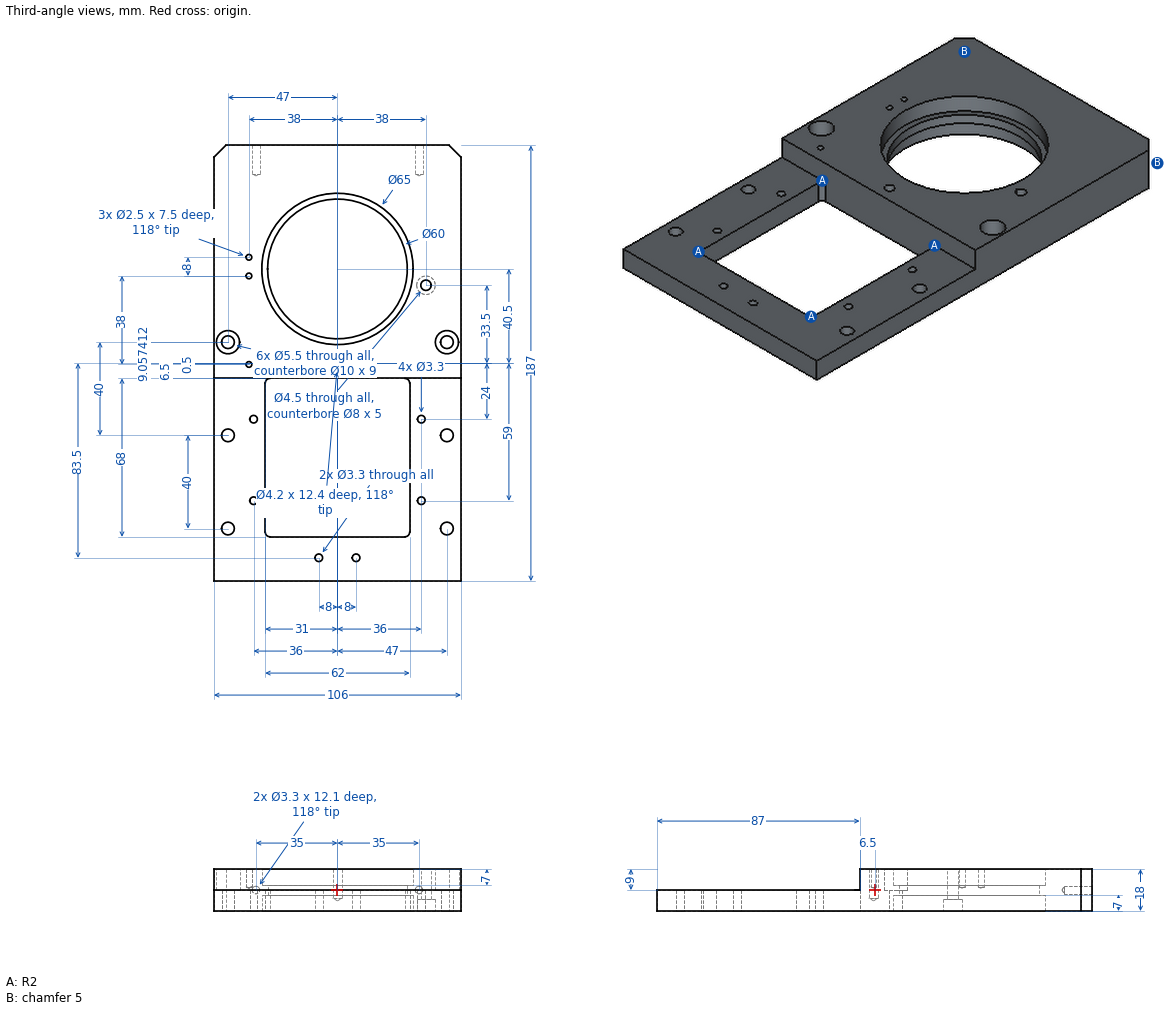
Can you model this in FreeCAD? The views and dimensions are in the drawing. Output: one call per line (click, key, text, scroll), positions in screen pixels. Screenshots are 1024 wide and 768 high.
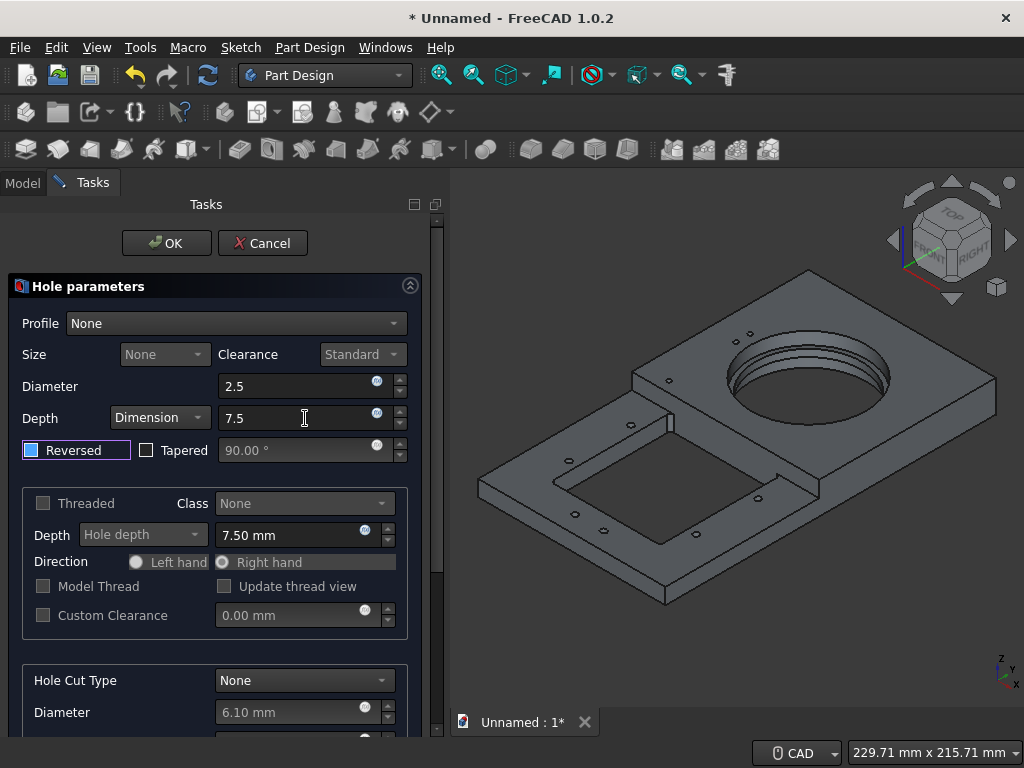
click(167, 243)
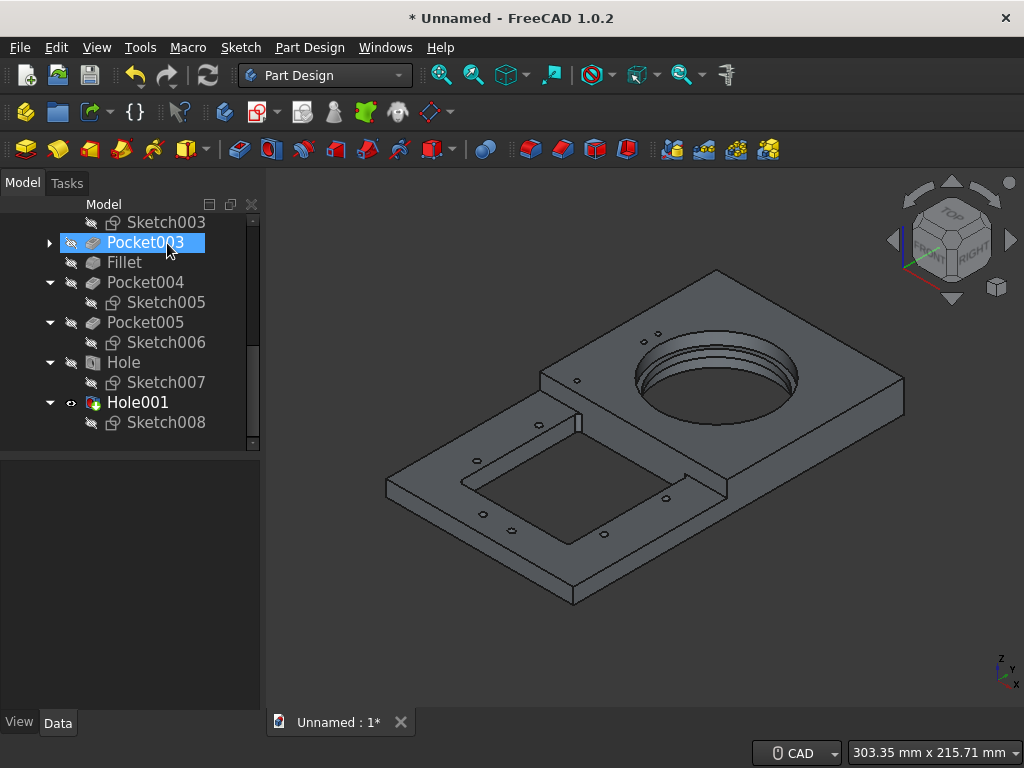
key(2)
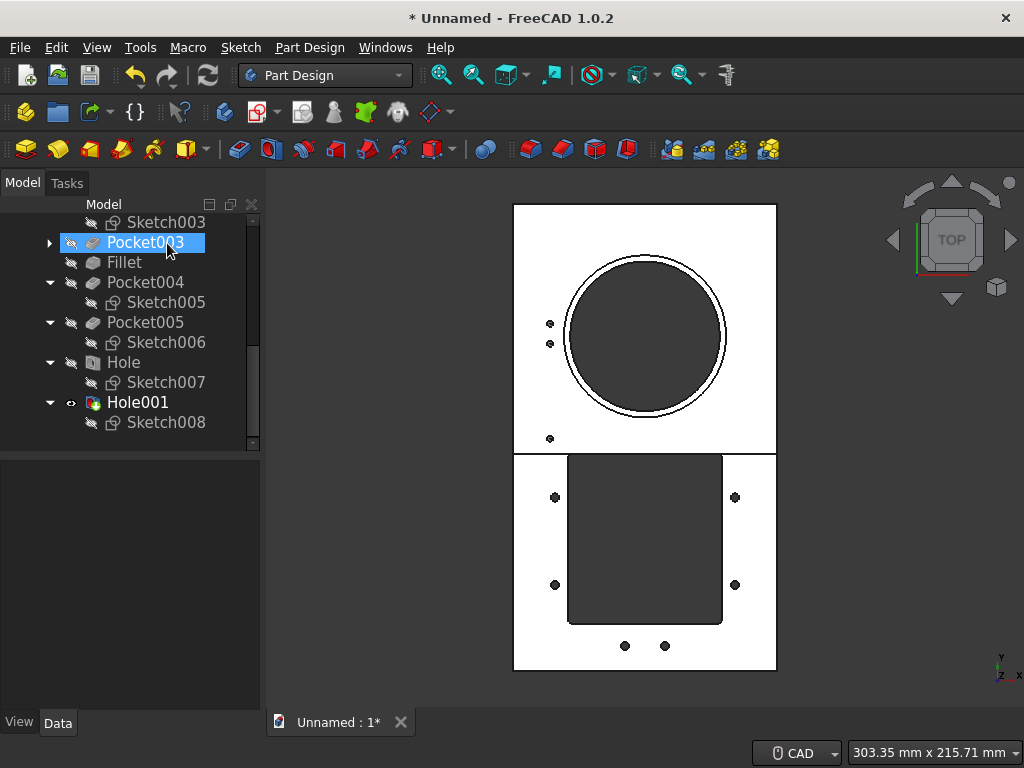
key(0)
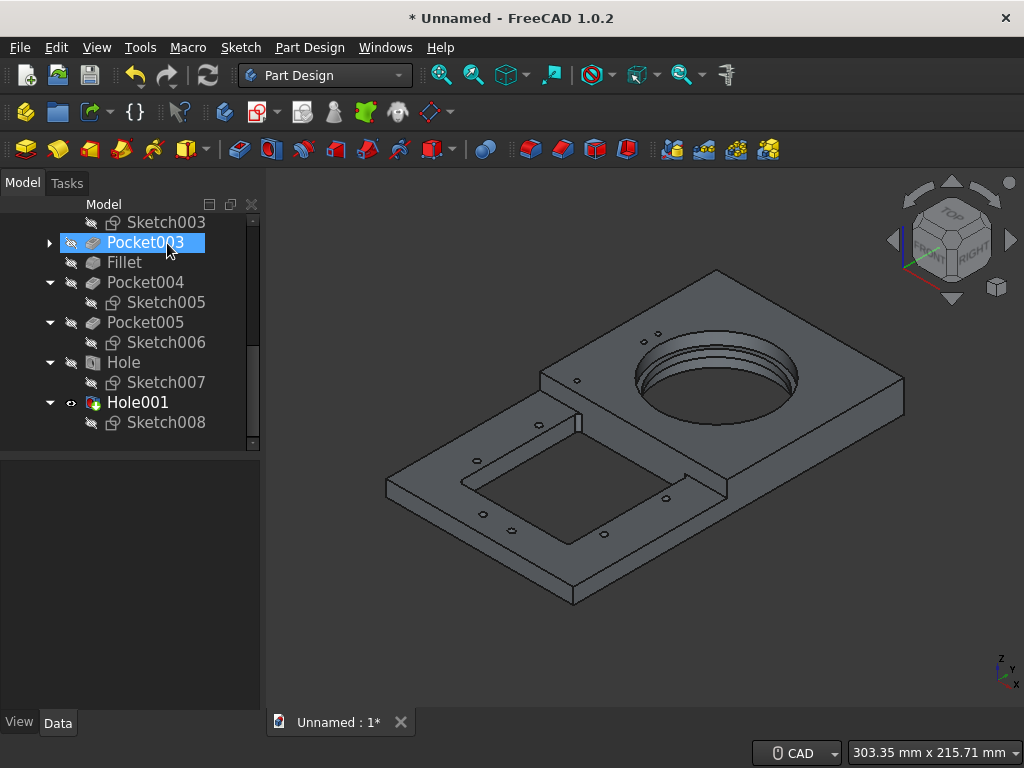
key(1)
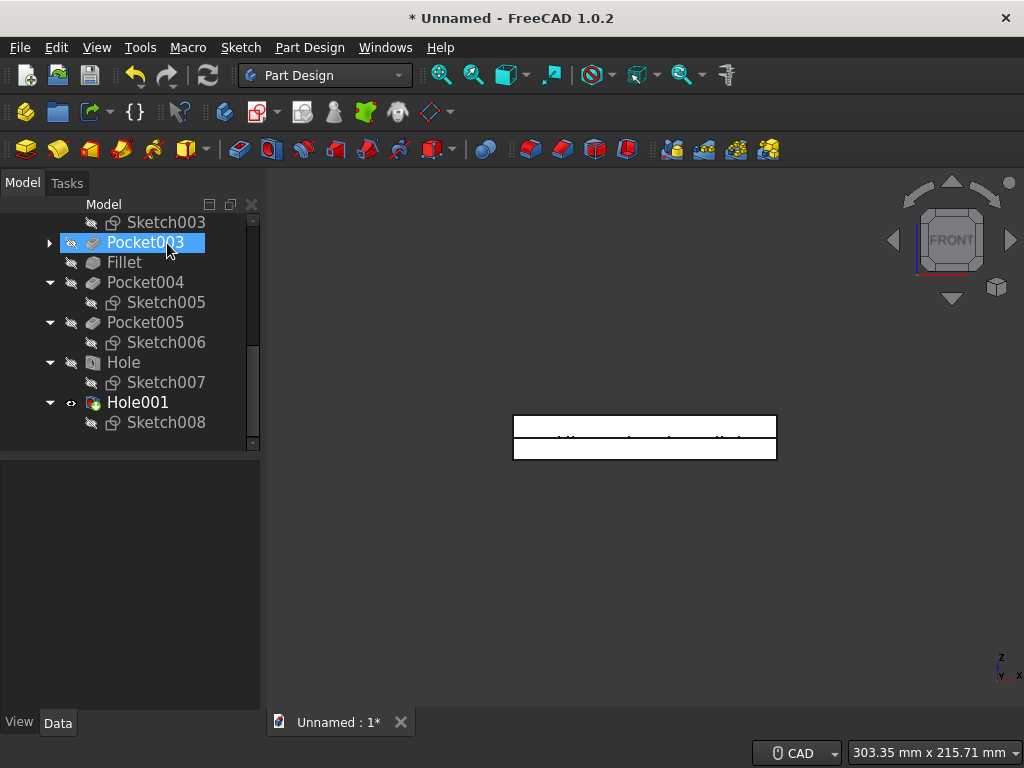
click(442, 76)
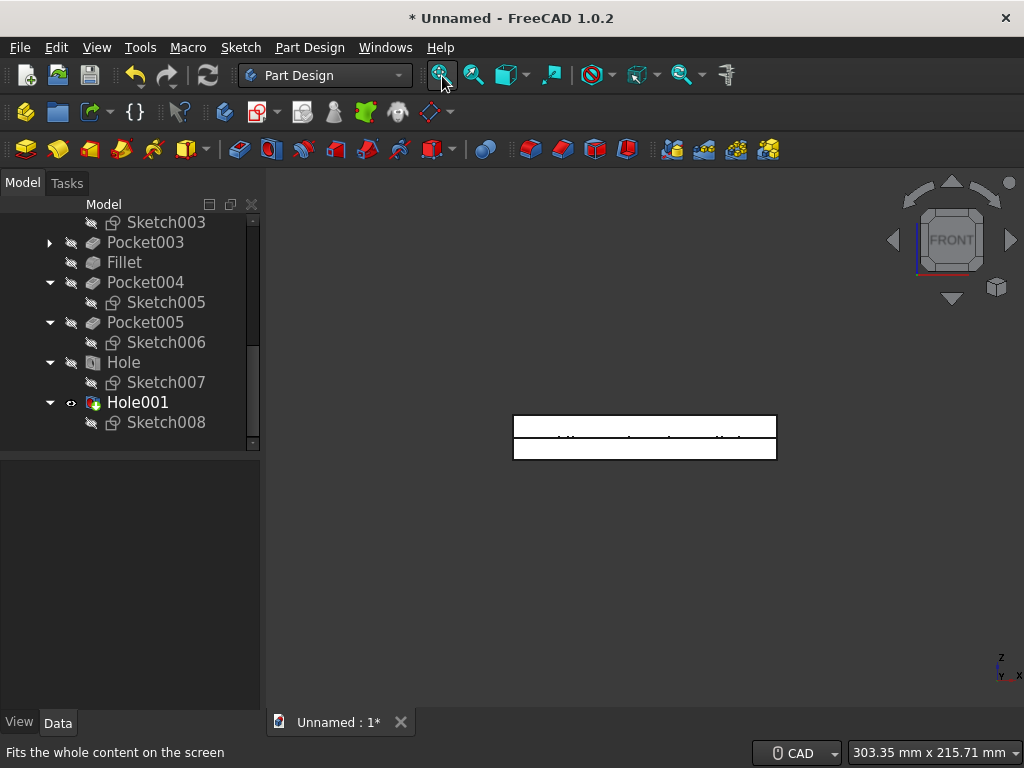
key(3)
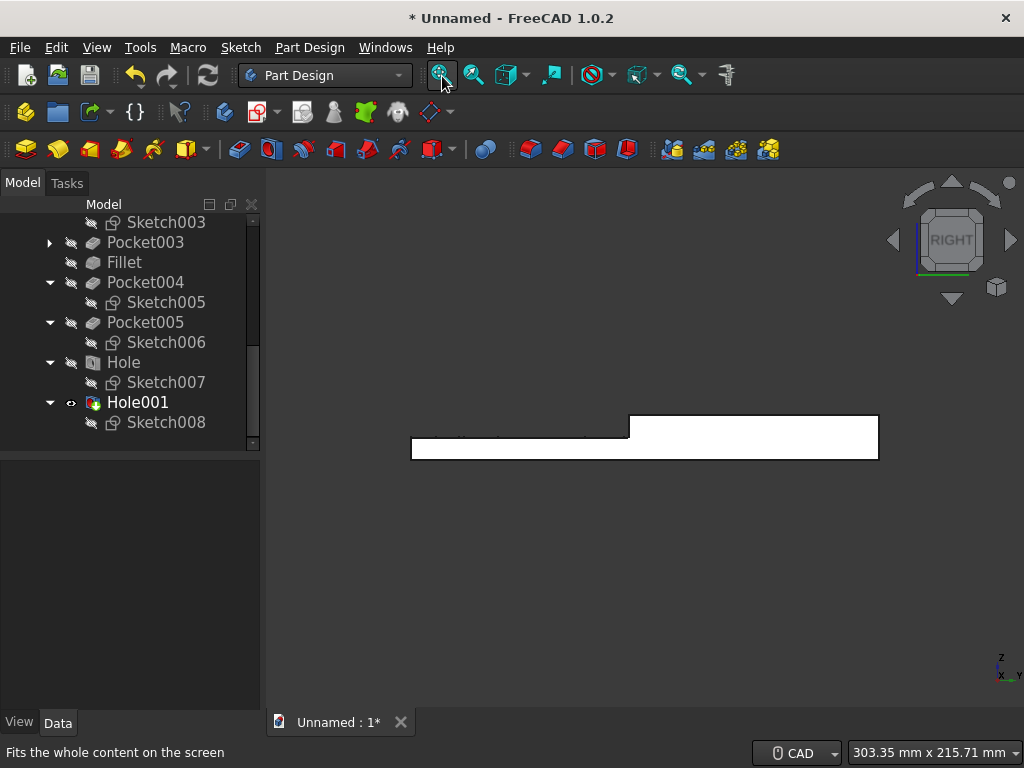
click(879, 436)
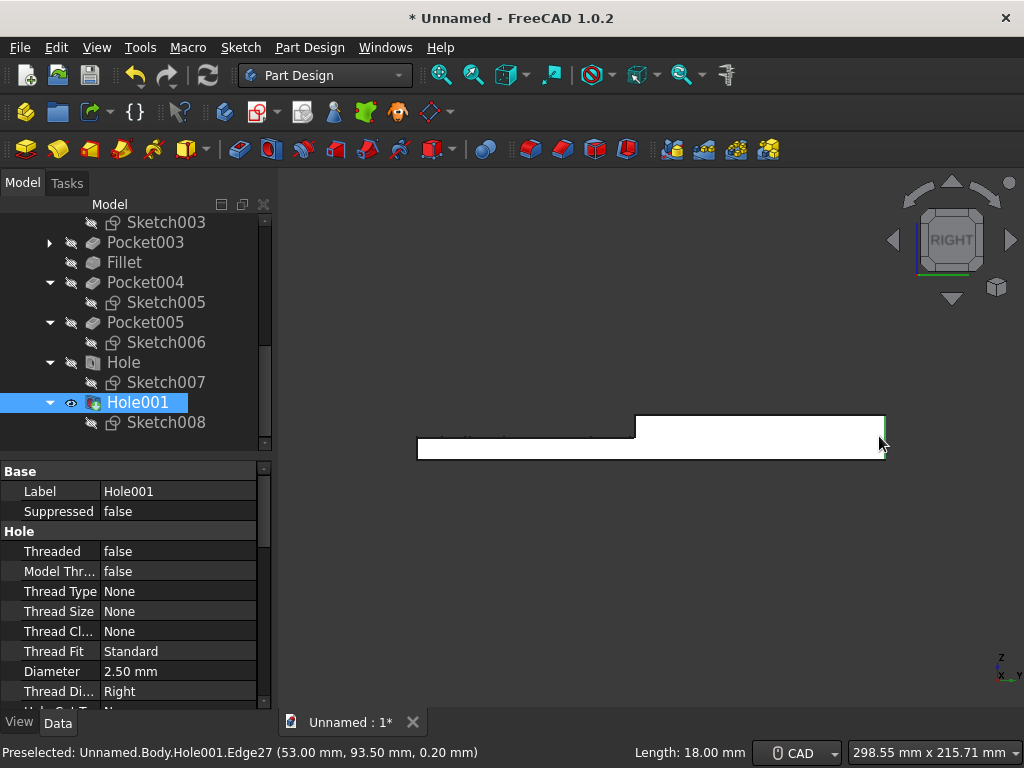
key(5)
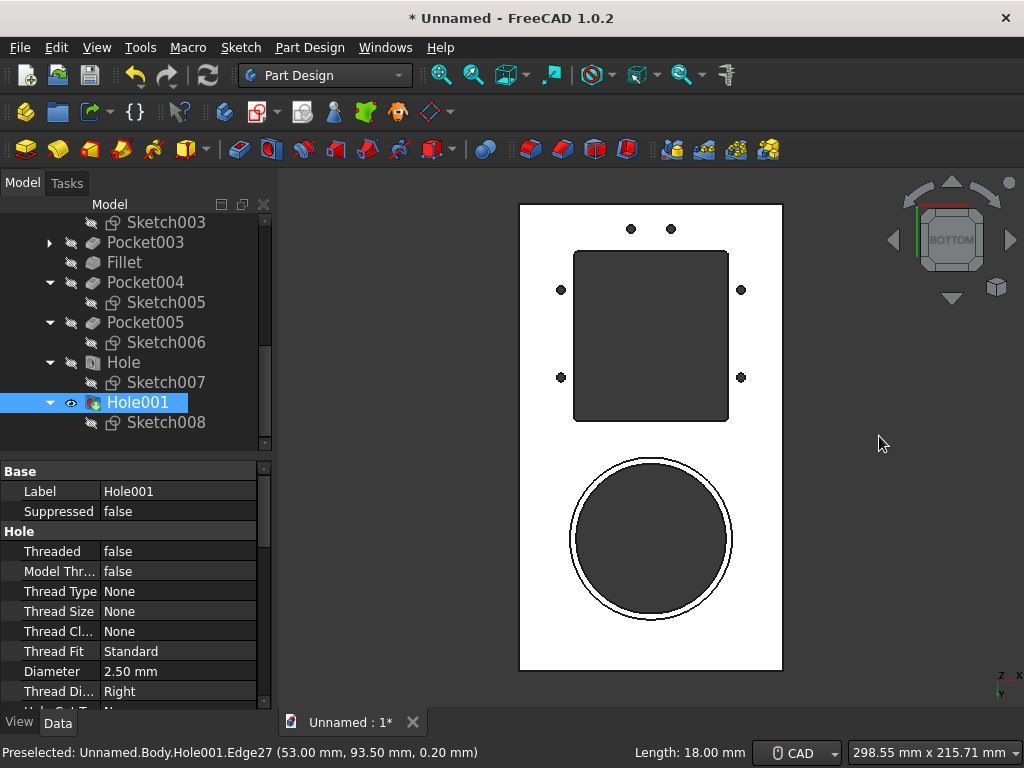
key(4)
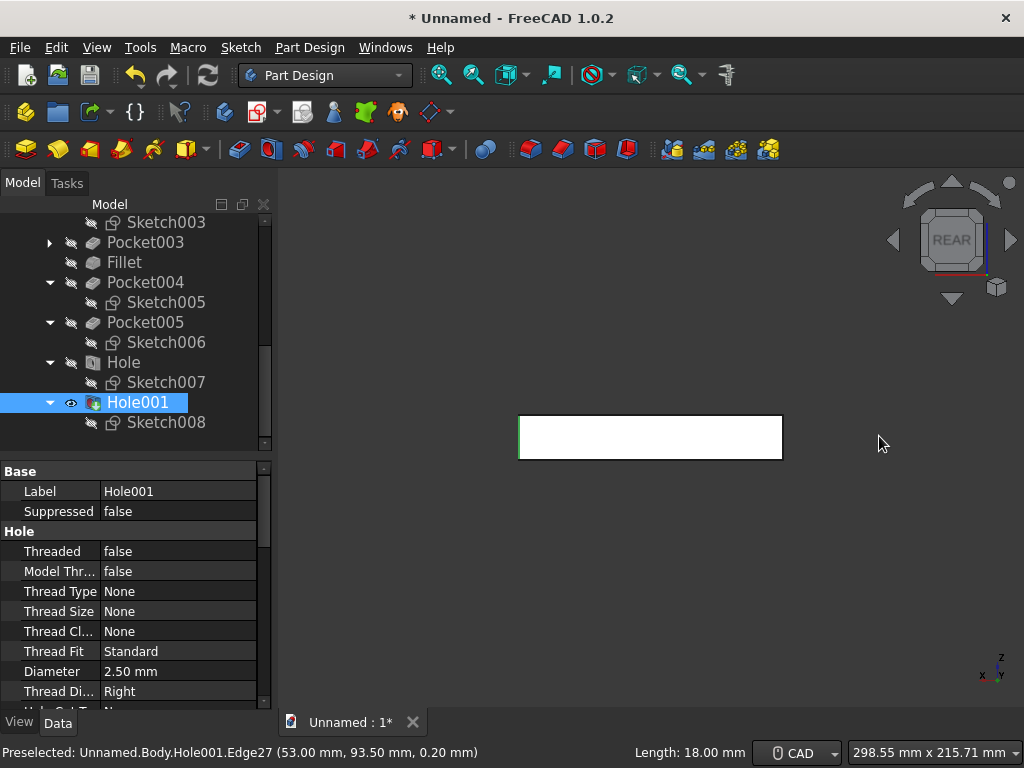
click(442, 76)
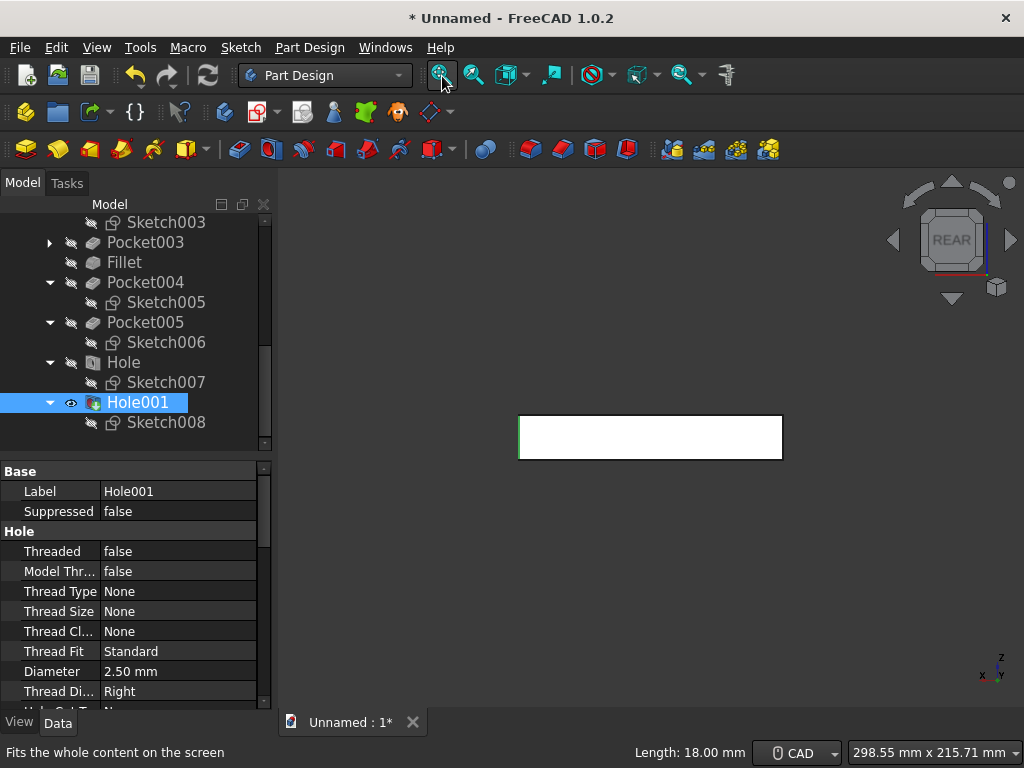
click(783, 437, ctrl)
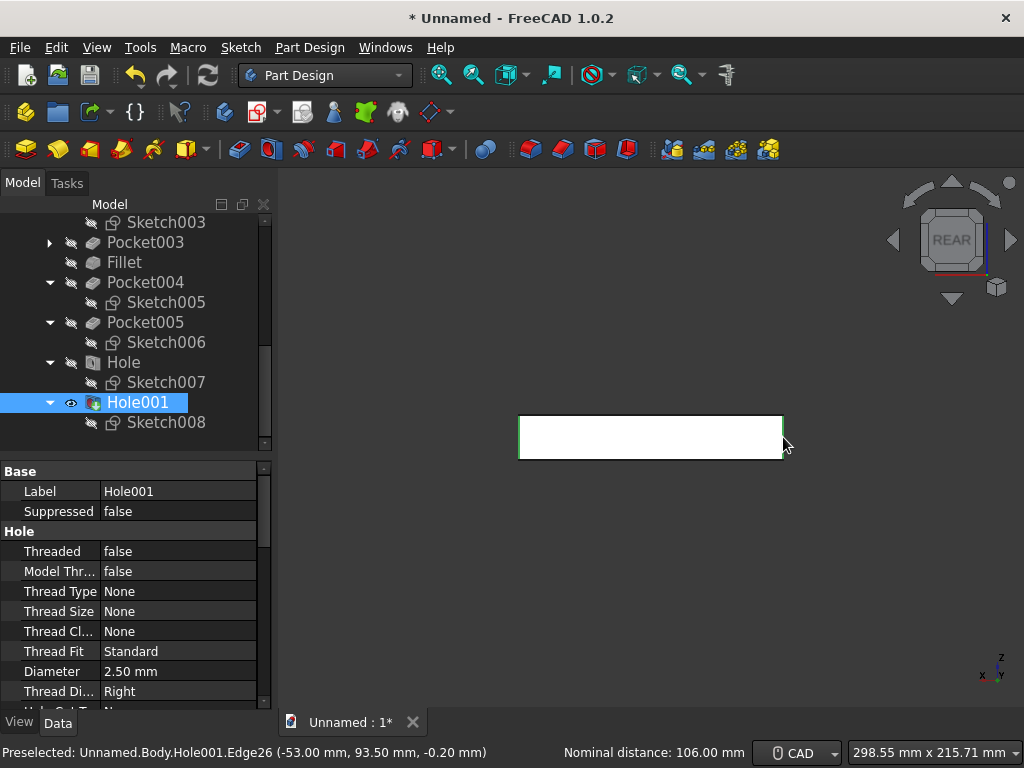
click(564, 150)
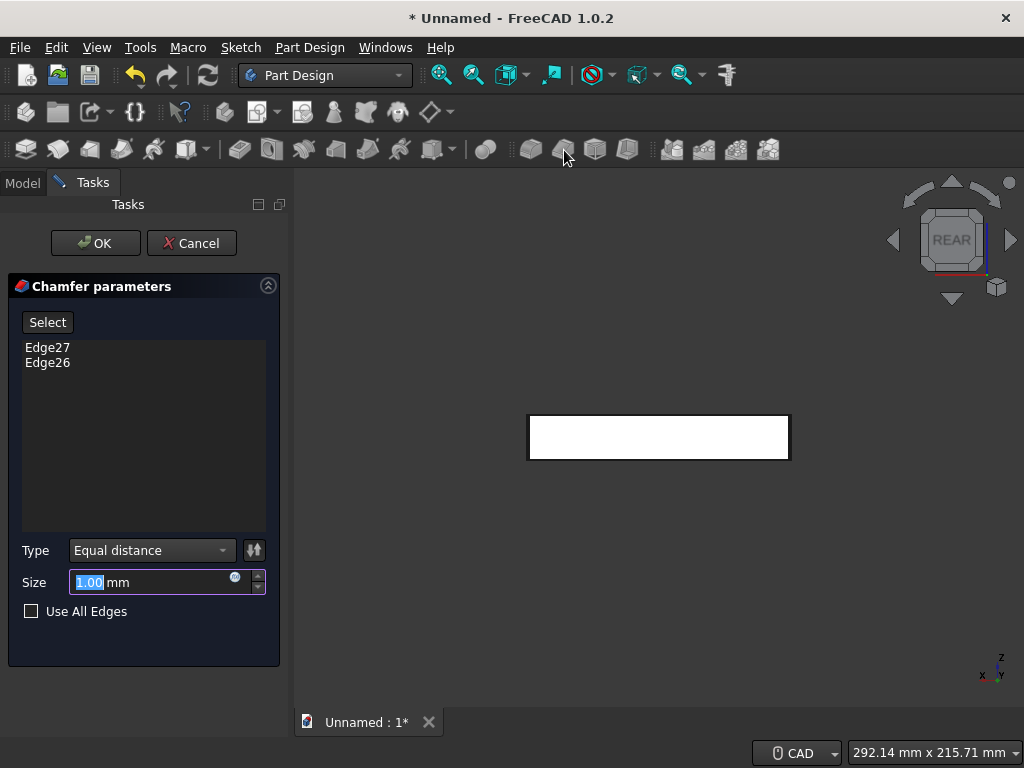
text(5)
key(Tab)